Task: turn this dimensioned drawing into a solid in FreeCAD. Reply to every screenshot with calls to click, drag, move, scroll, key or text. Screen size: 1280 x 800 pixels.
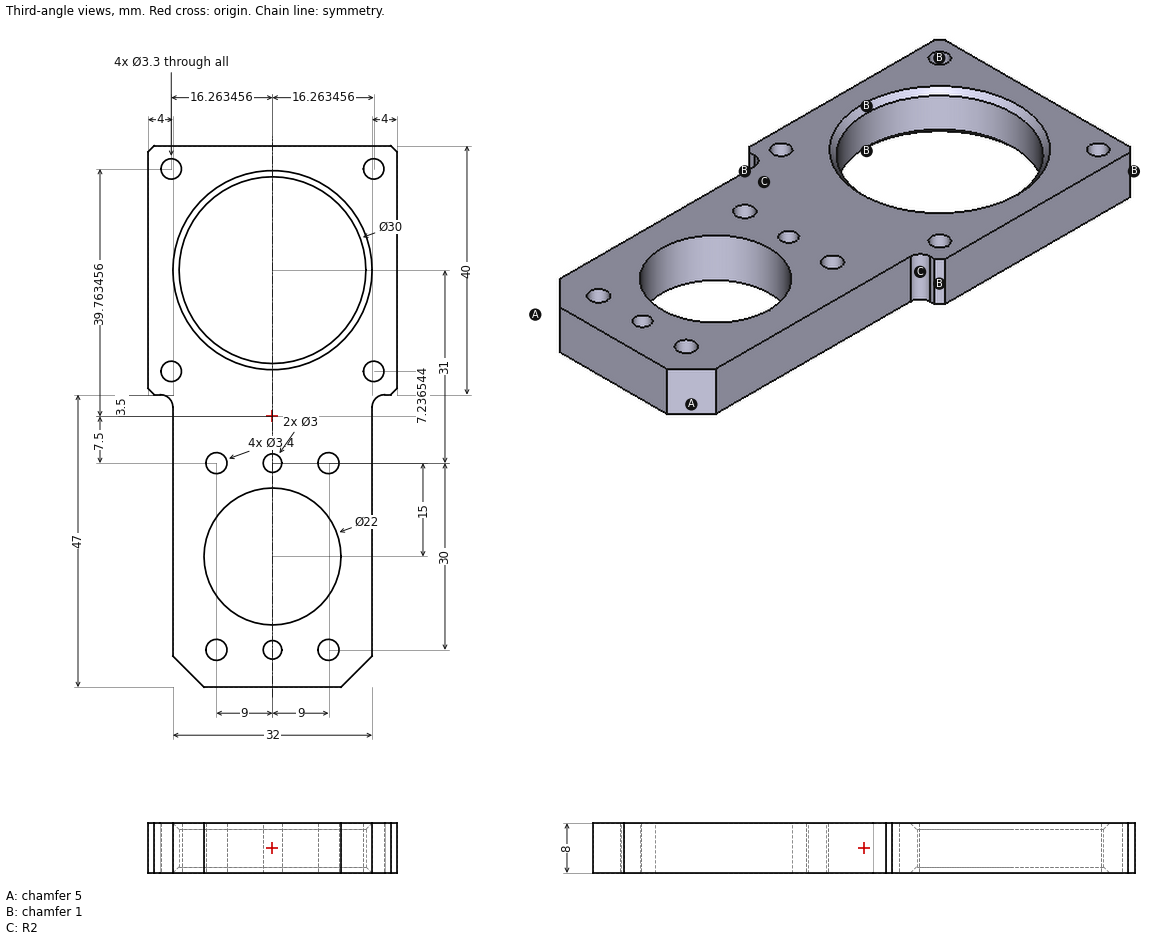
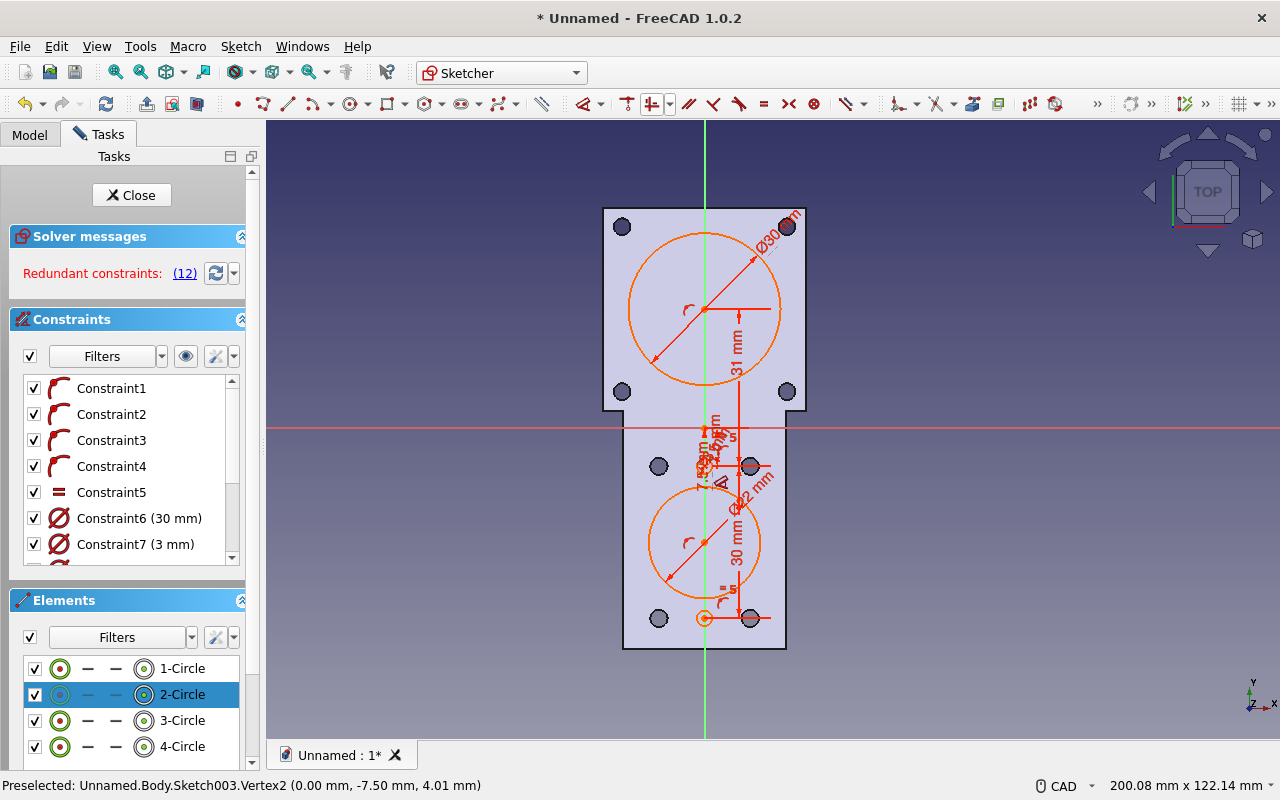
click(705, 543)
click(739, 522)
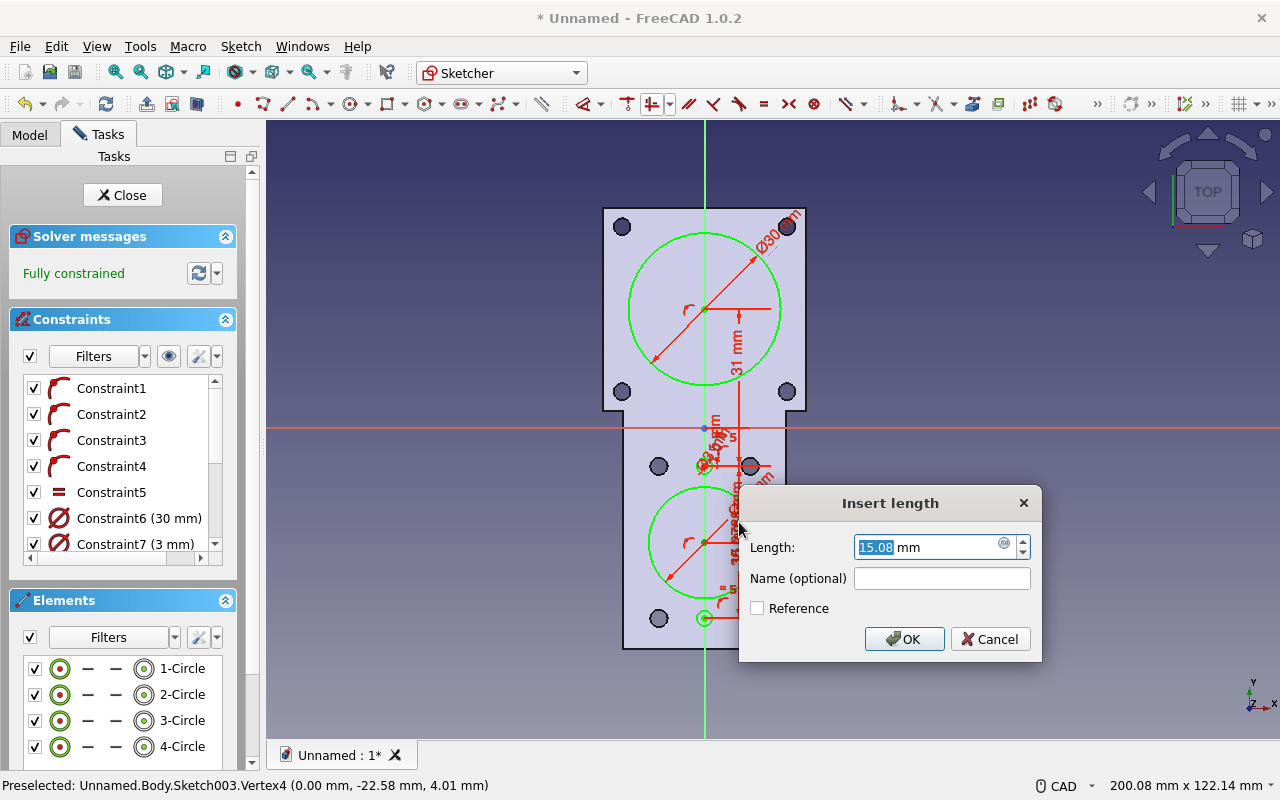
text(15)
key(Return)
key(Escape)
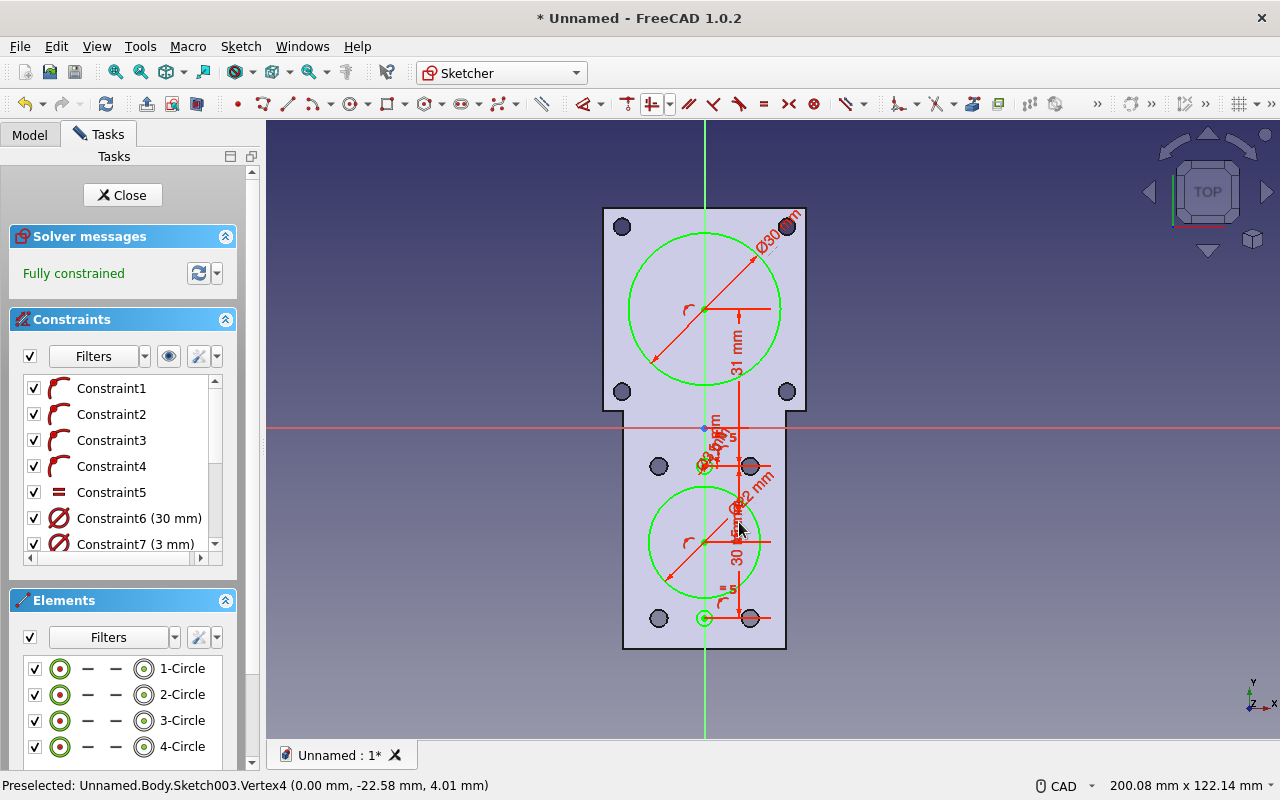
click(123, 195)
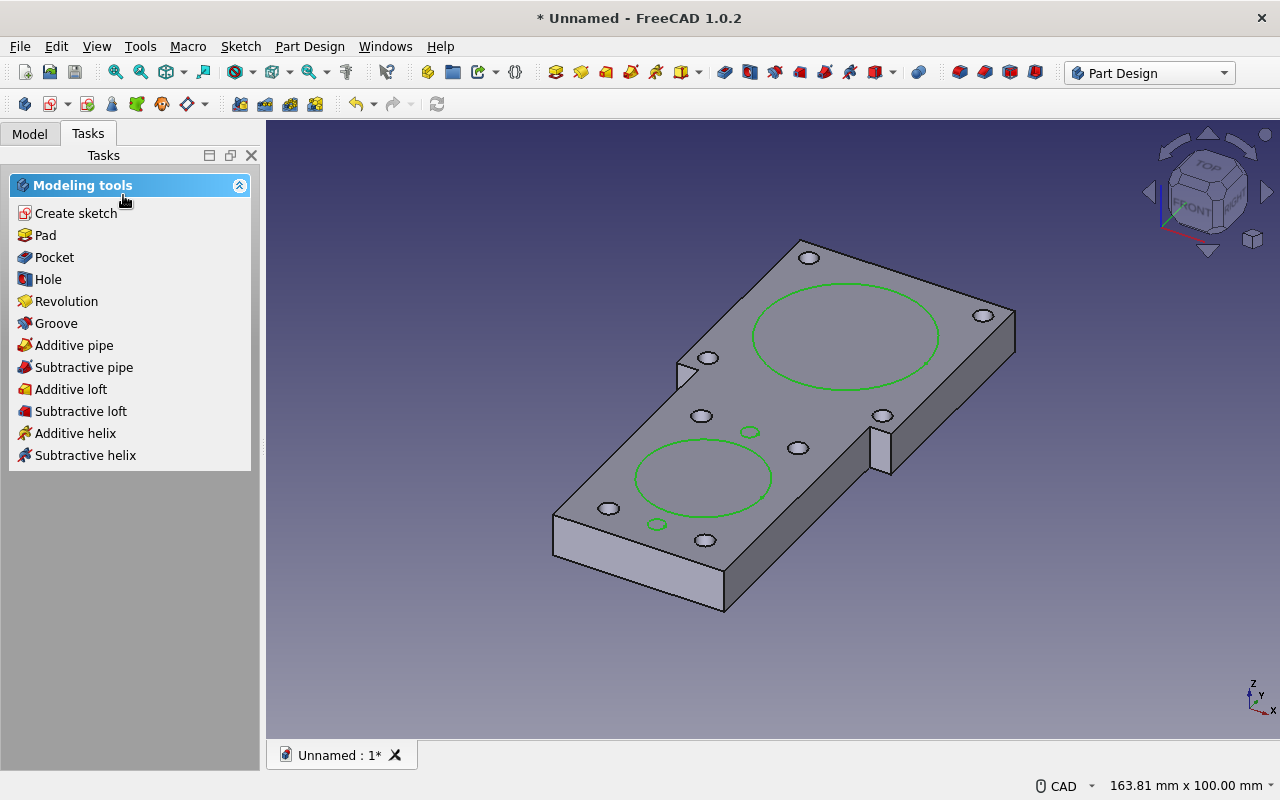
click(725, 72)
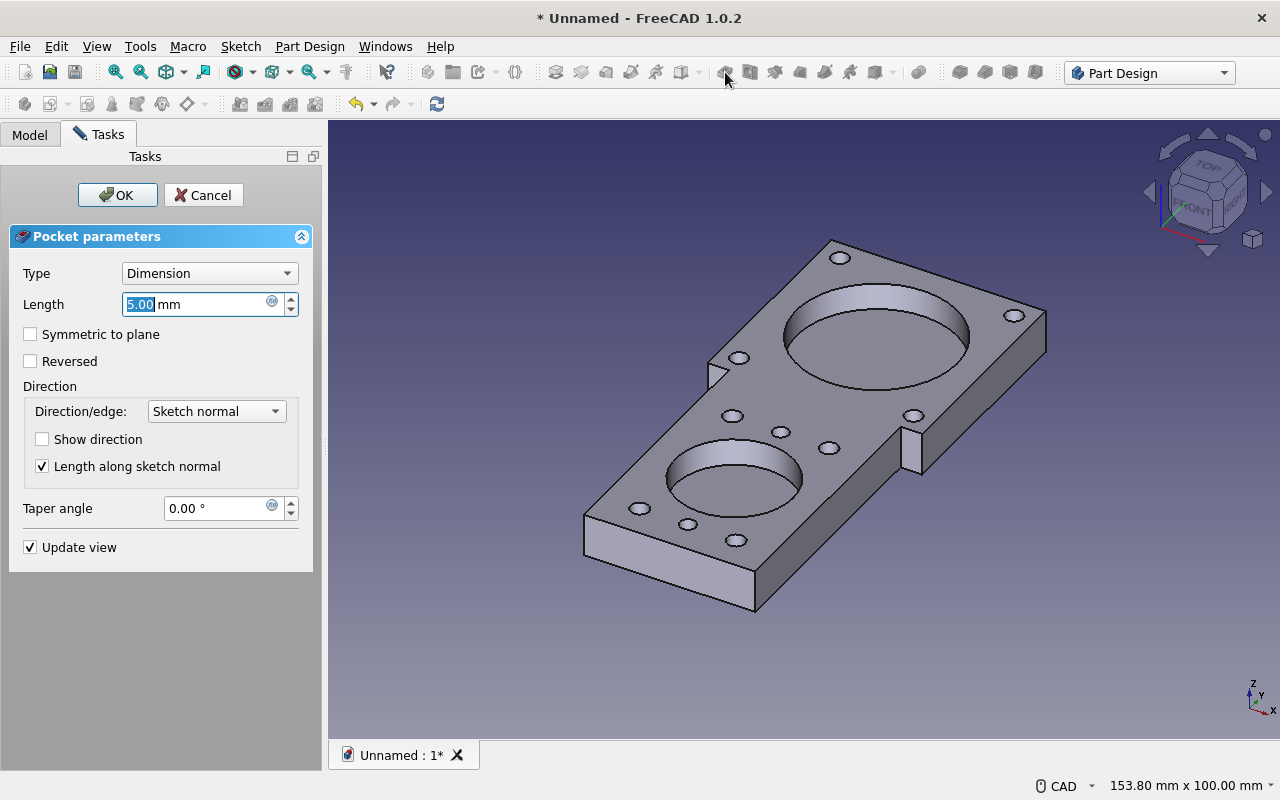
click(210, 274)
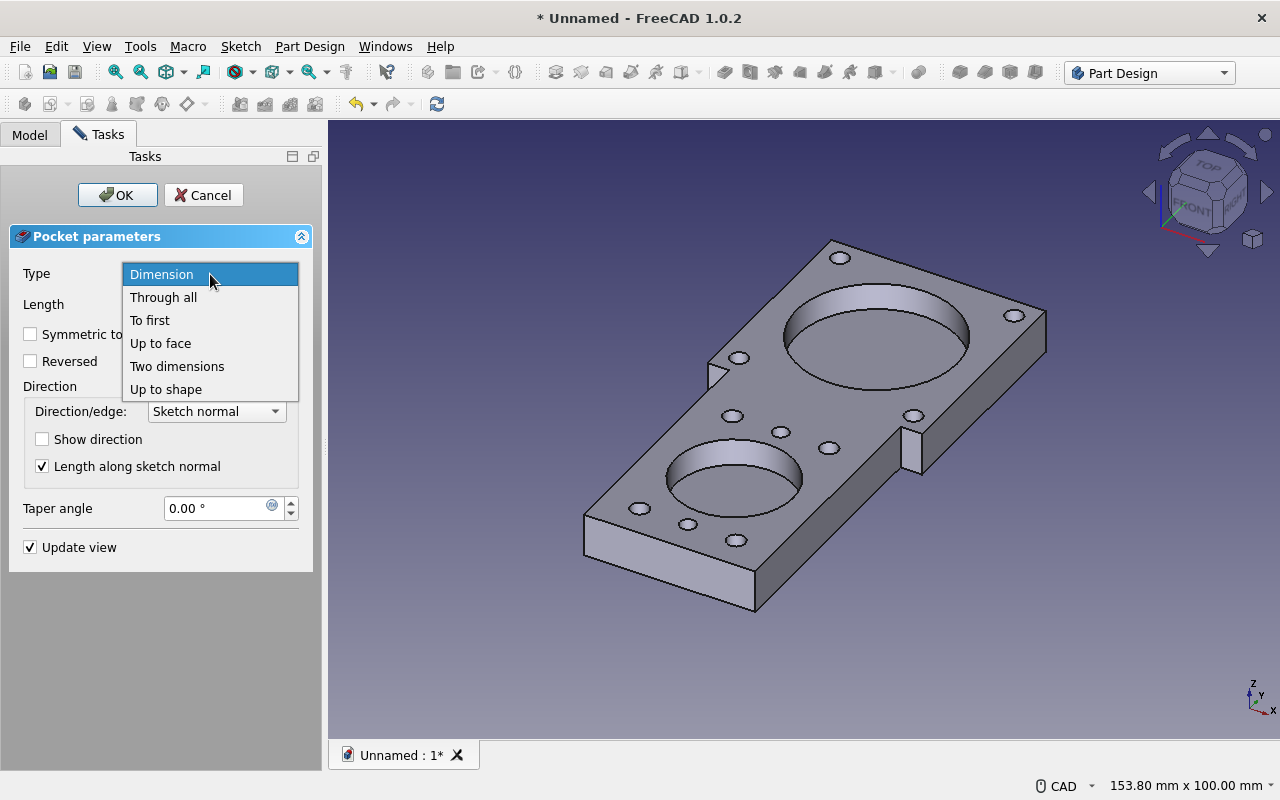
click(208, 298)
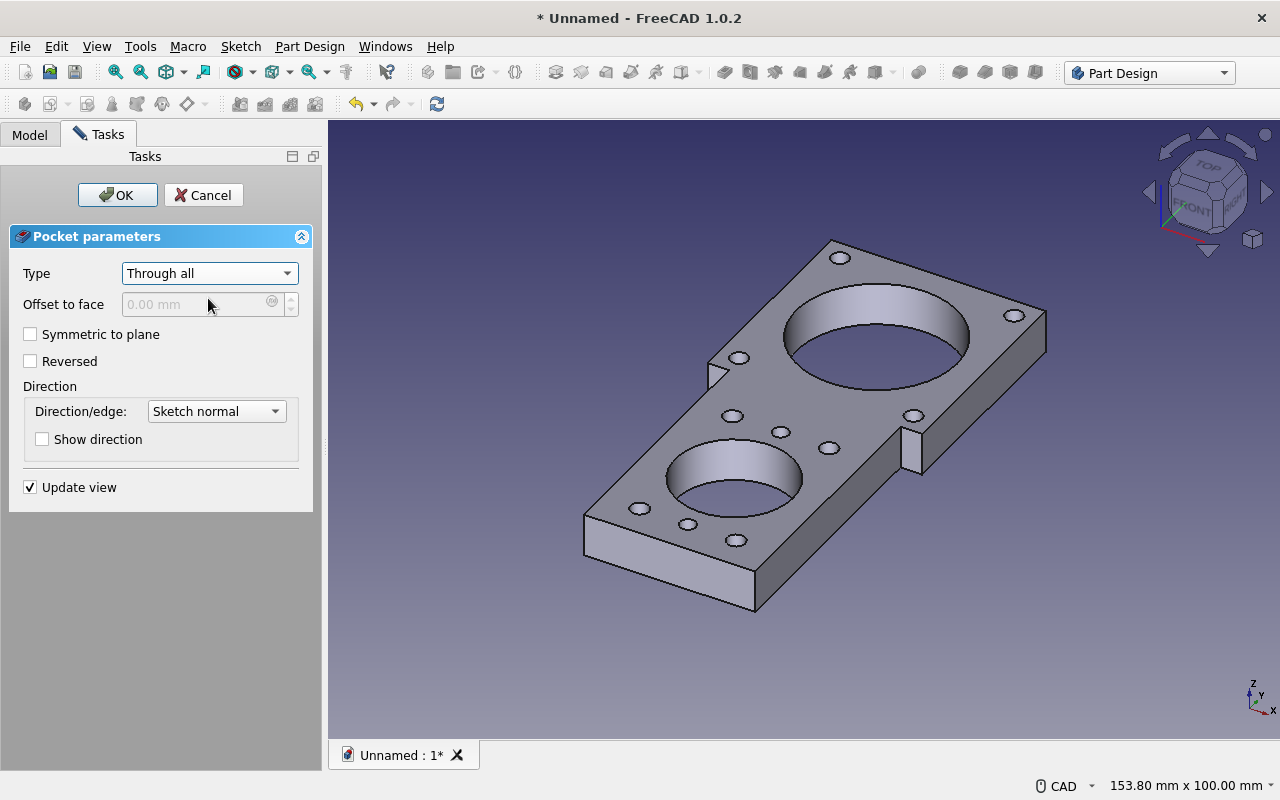
click(118, 195)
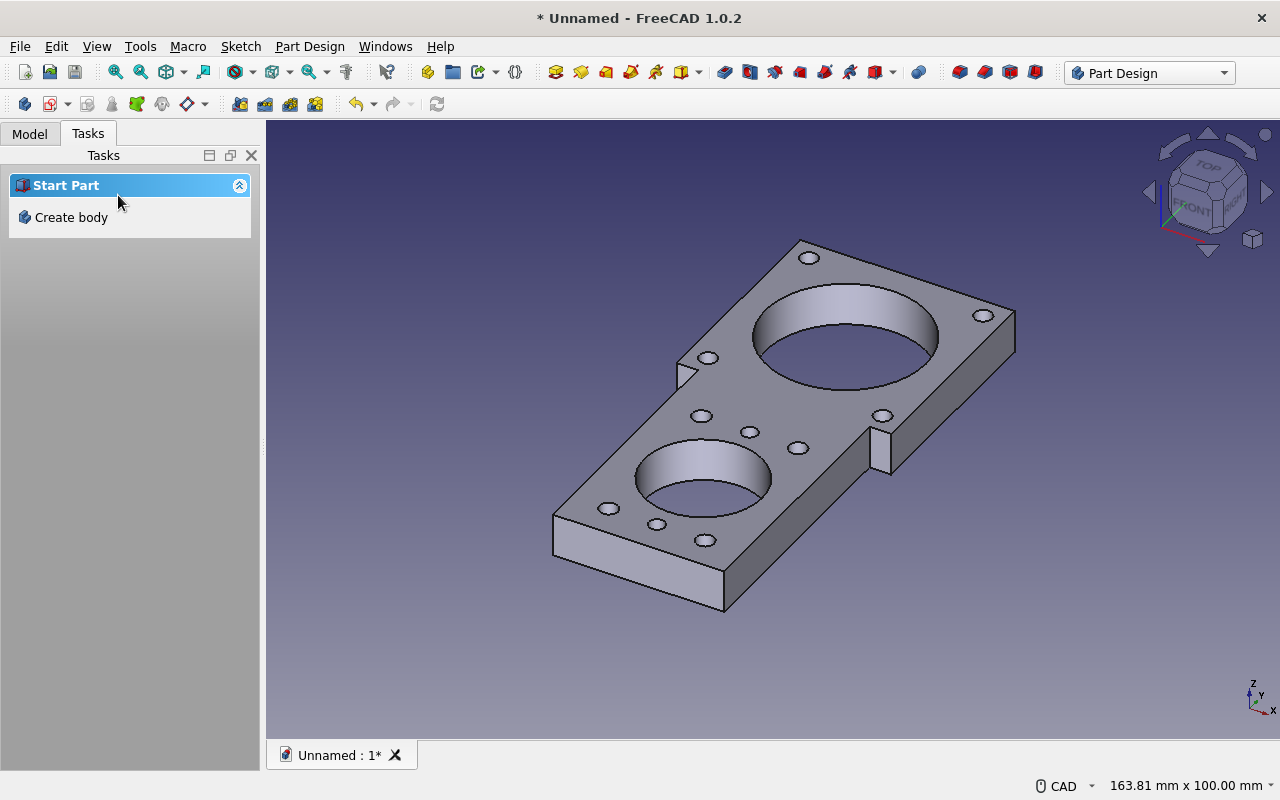
click(724, 591)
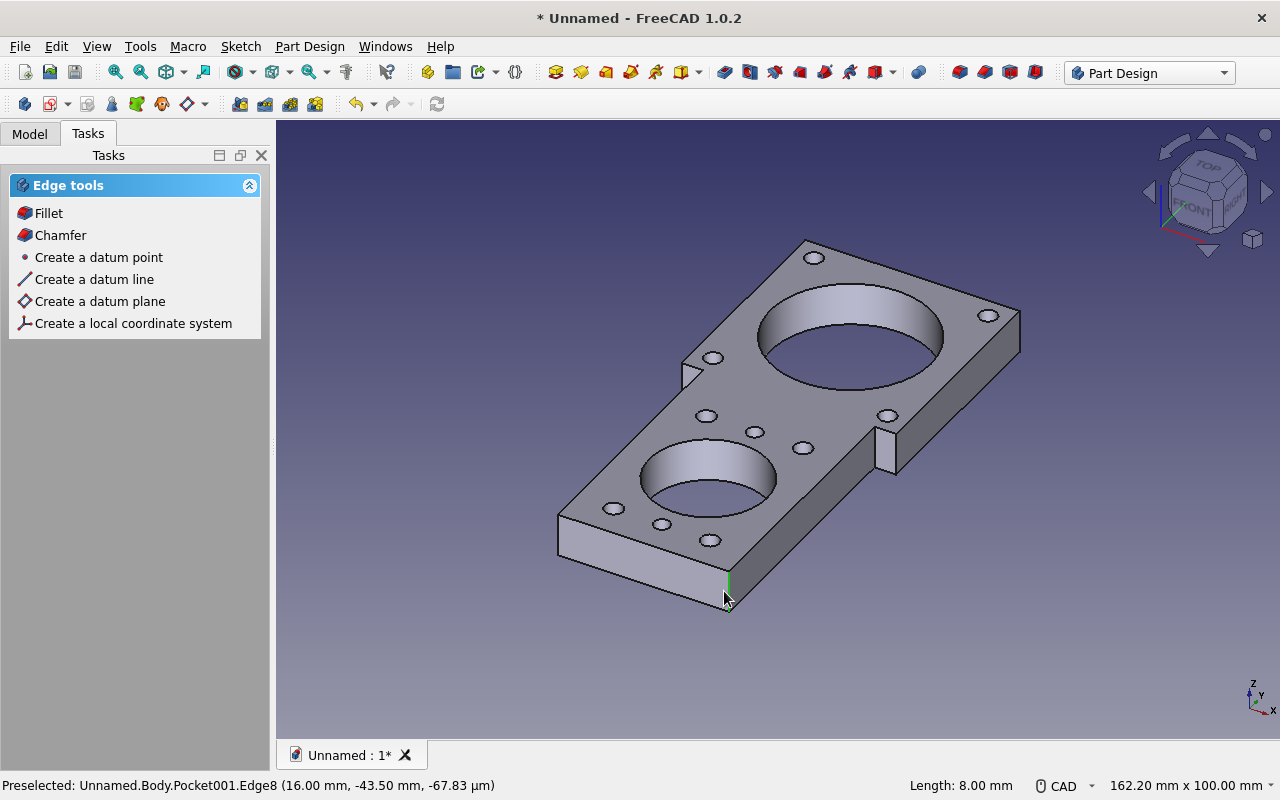
key(0)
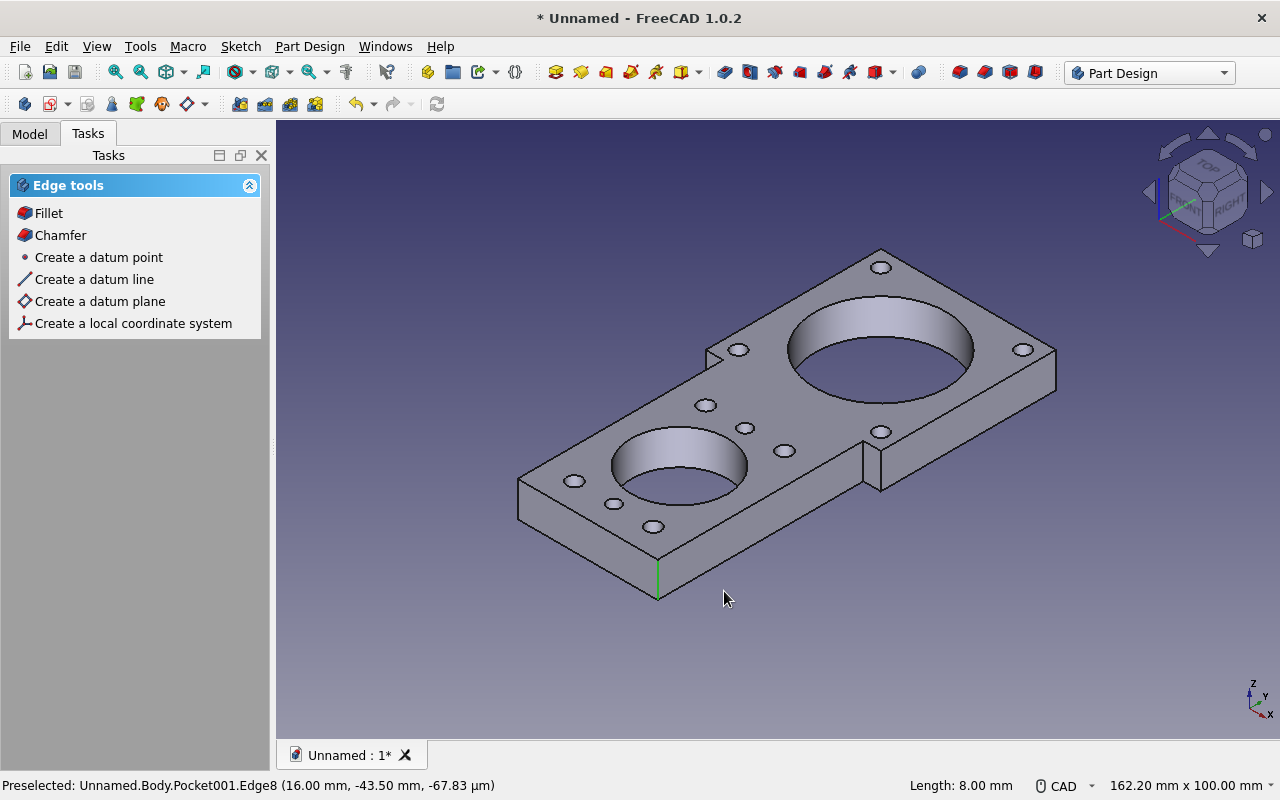
key(2)